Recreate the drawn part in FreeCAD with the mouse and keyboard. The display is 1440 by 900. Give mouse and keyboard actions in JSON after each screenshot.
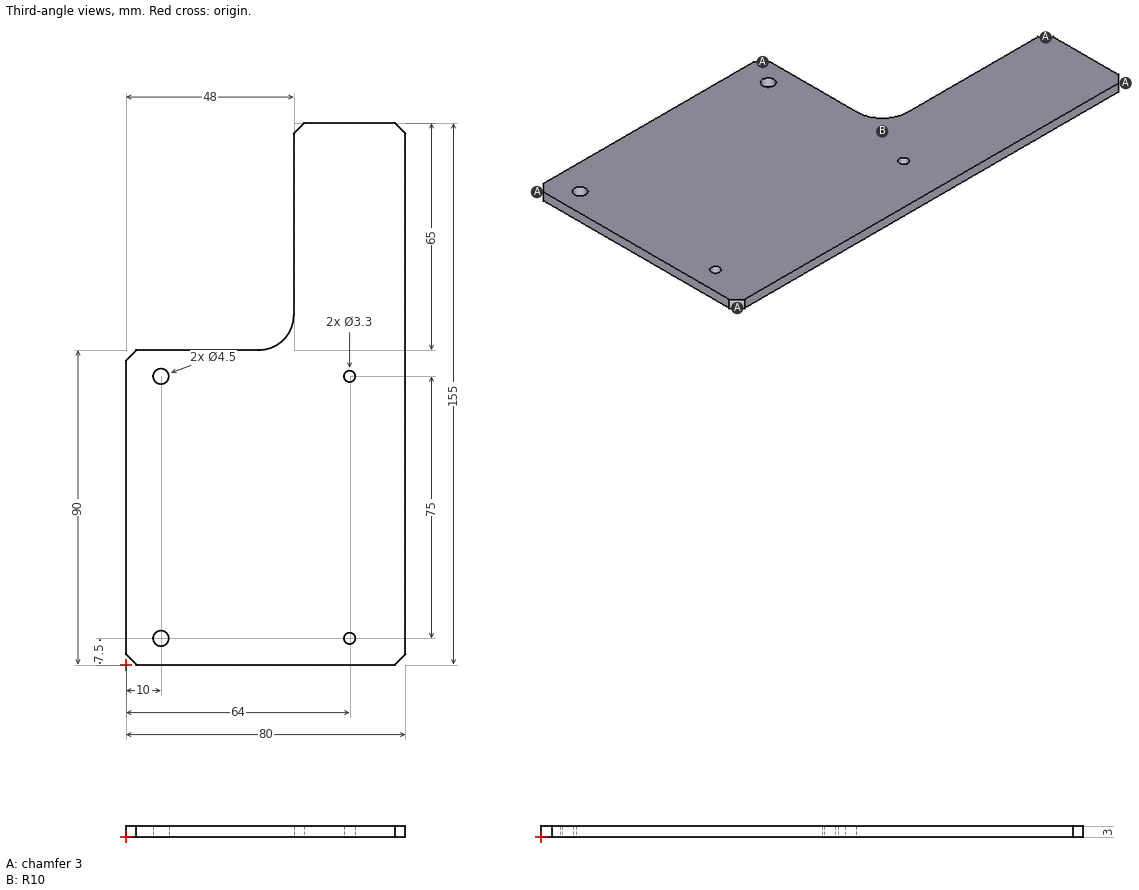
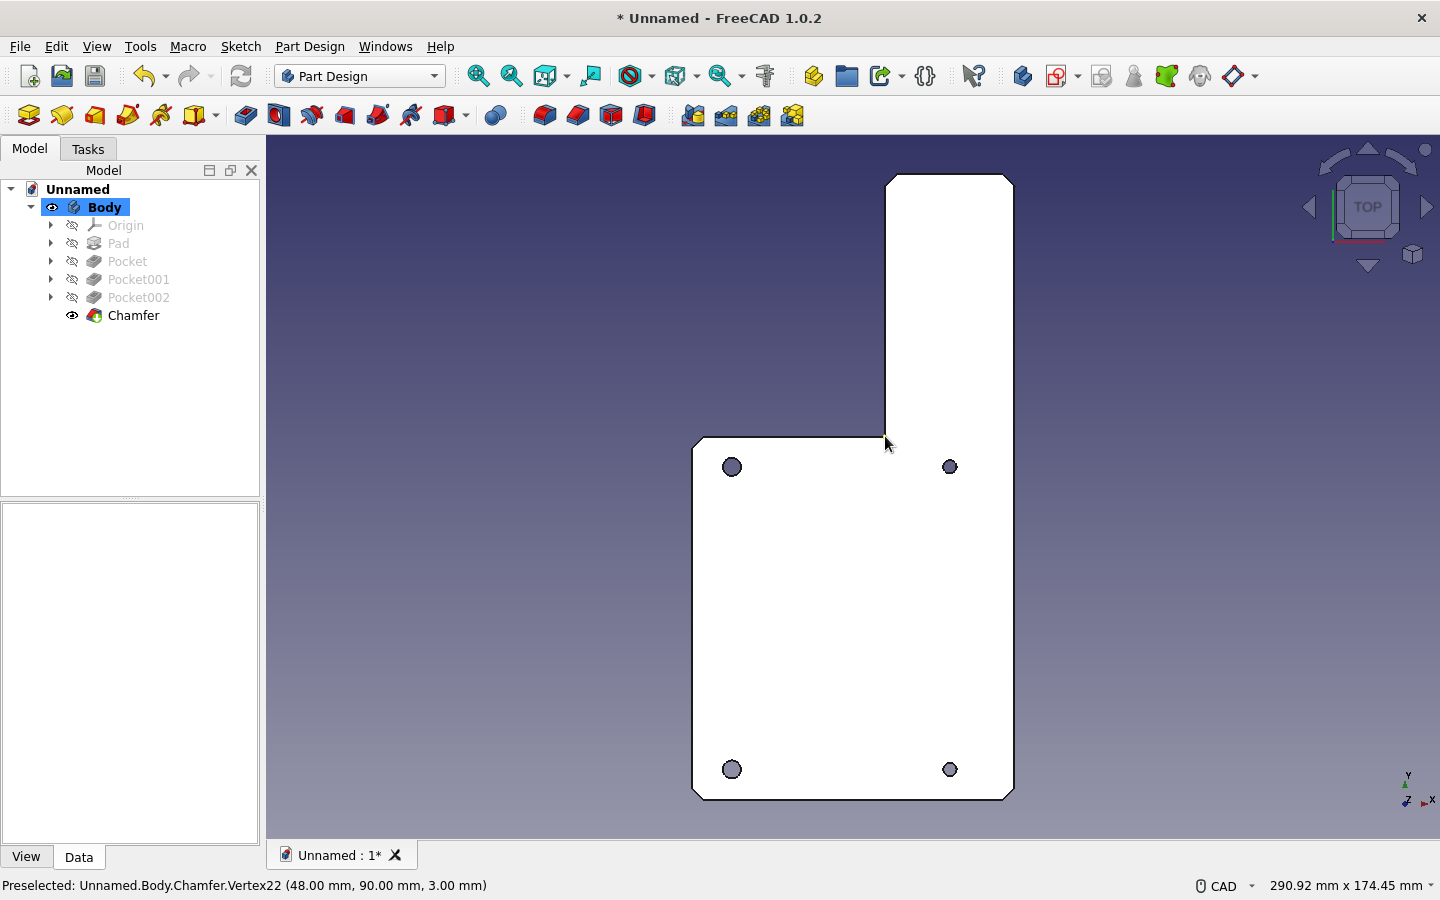
{"action": "key", "text": "1"}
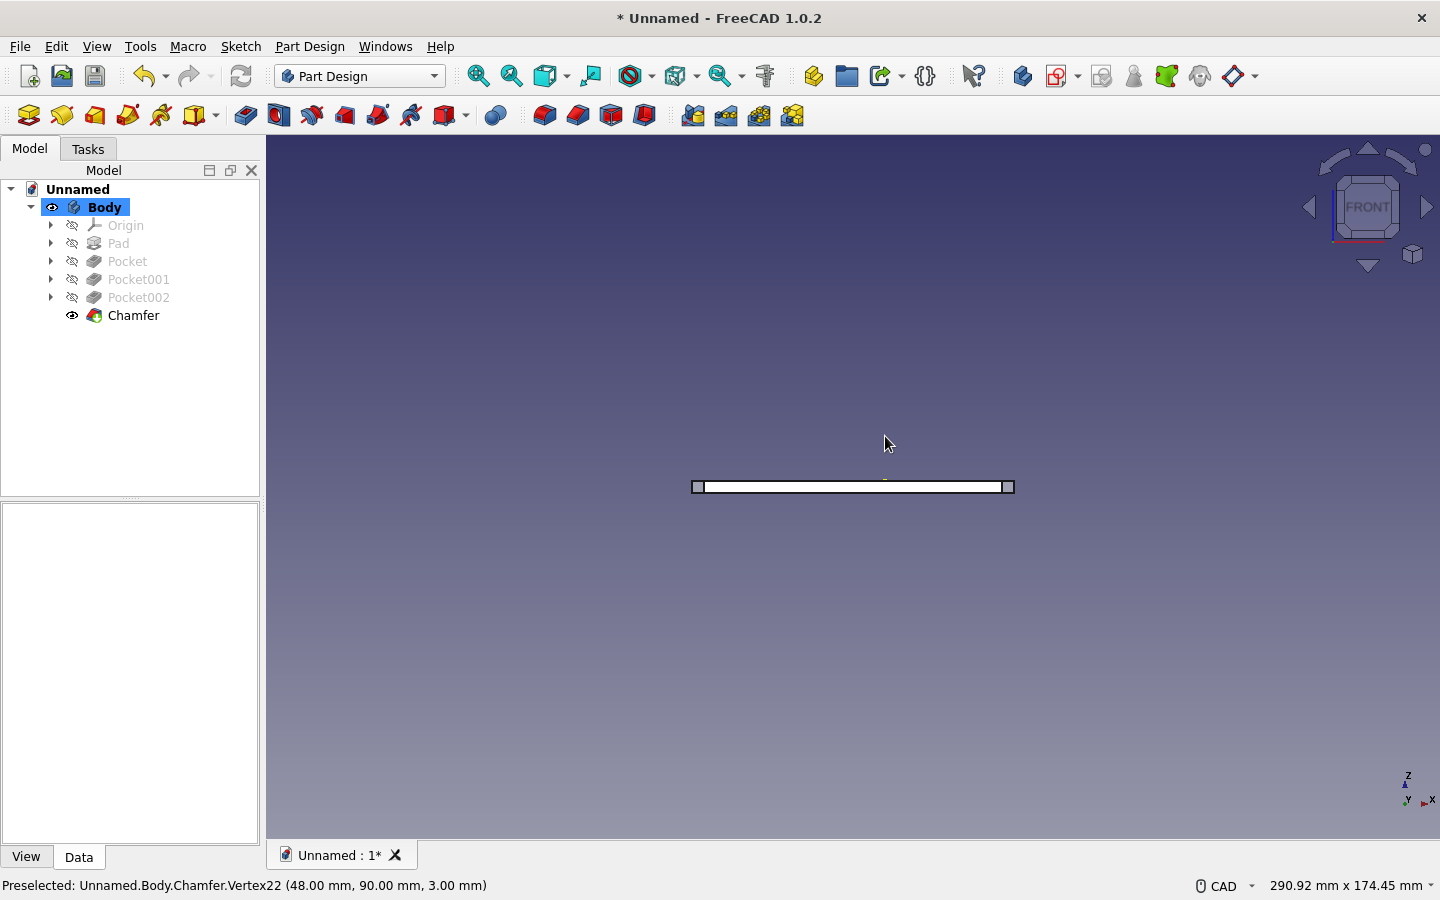
{"action": "key", "text": "v f"}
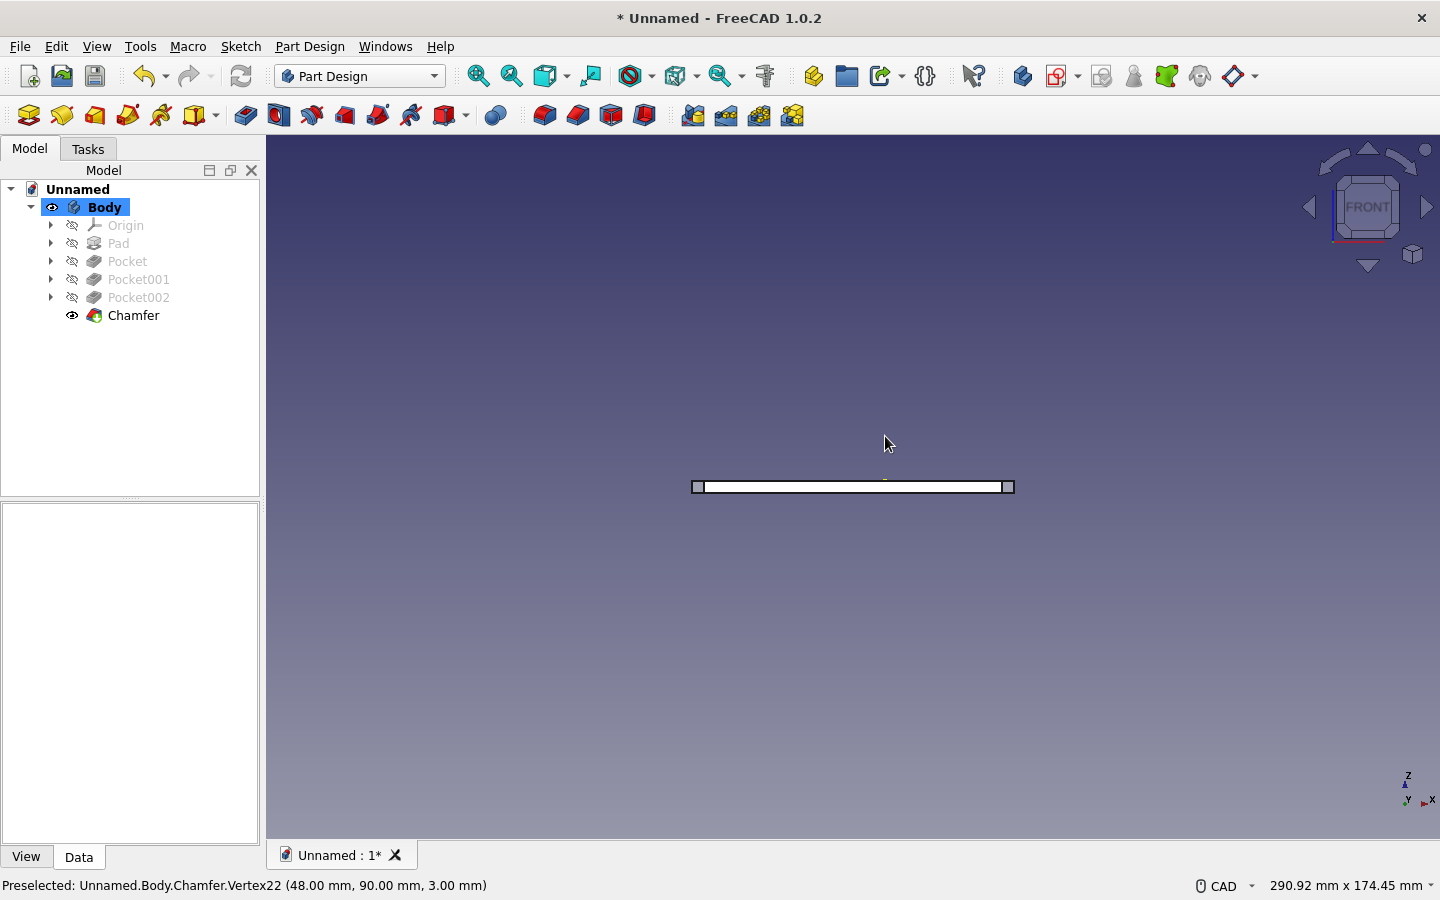
{"action": "scroll", "coordinate": [885, 486], "scroll_direction": "up", "scroll_amount": 6}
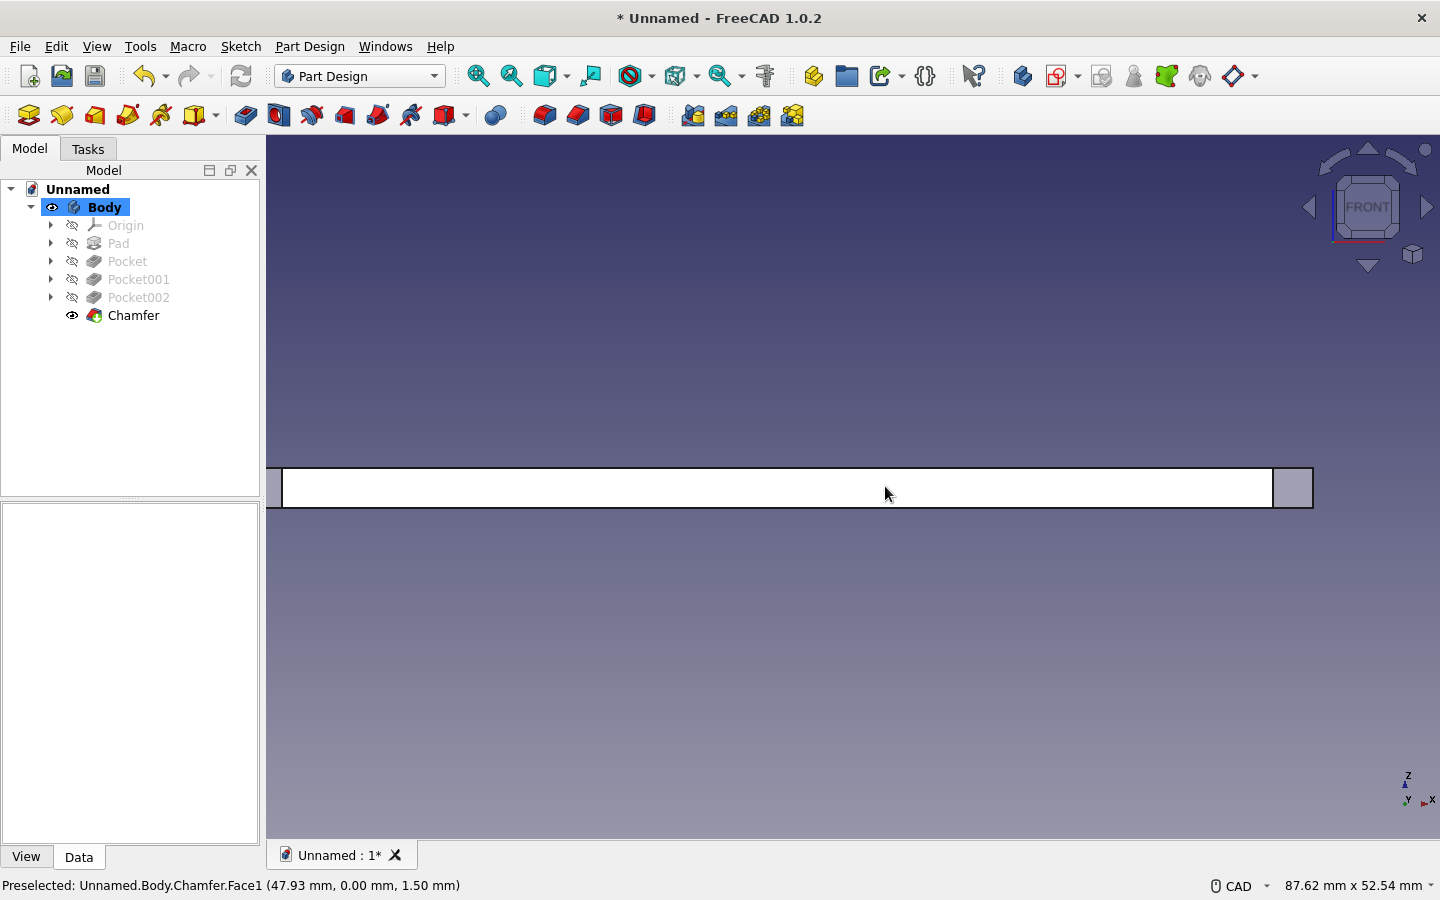
{"action": "left_click", "coordinate": [479, 76]}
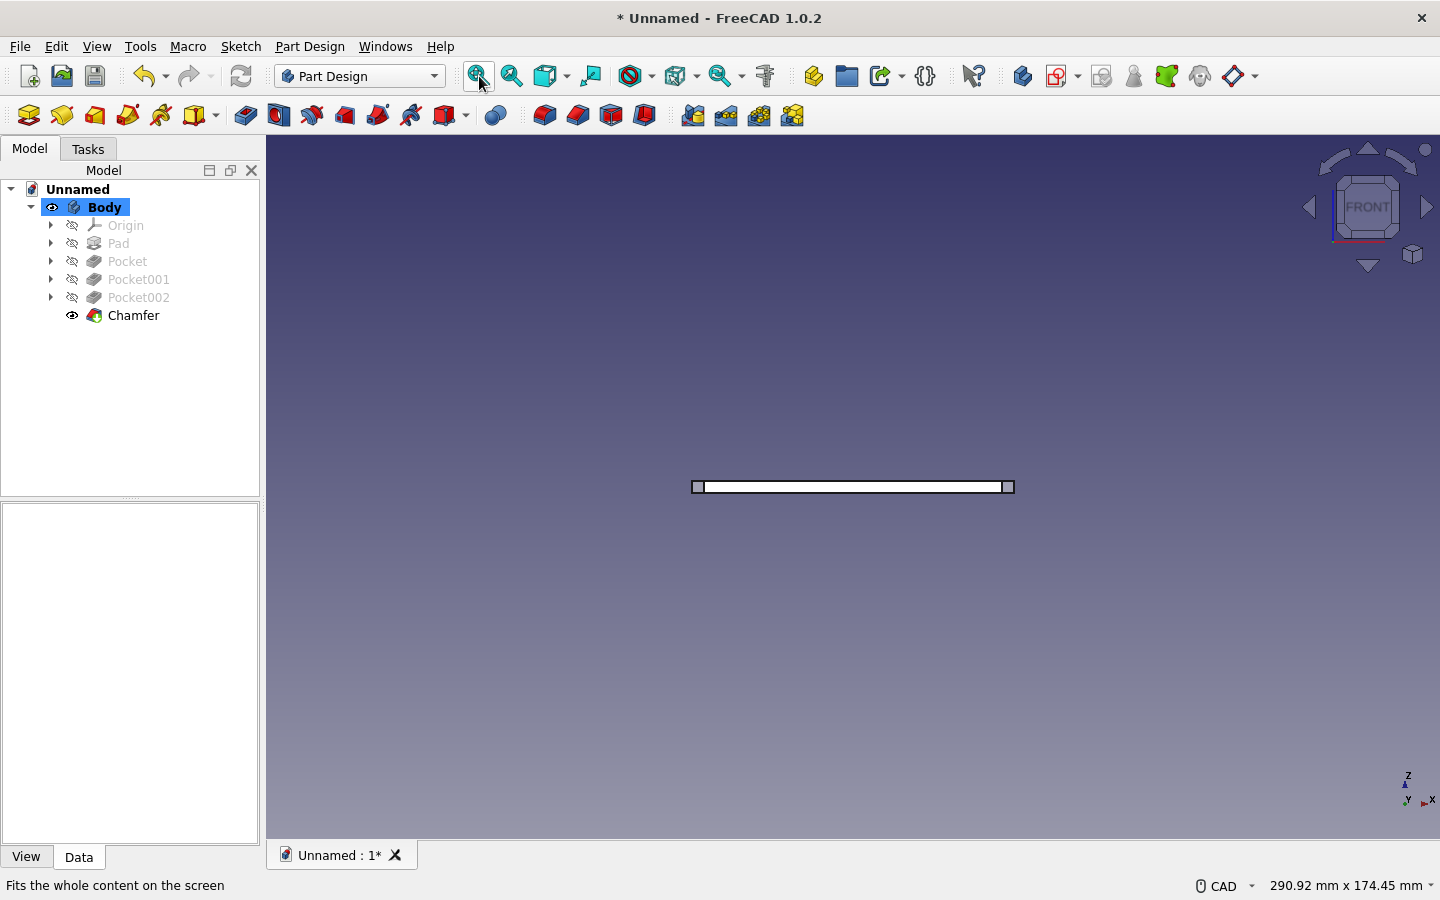
{"action": "key", "text": "3"}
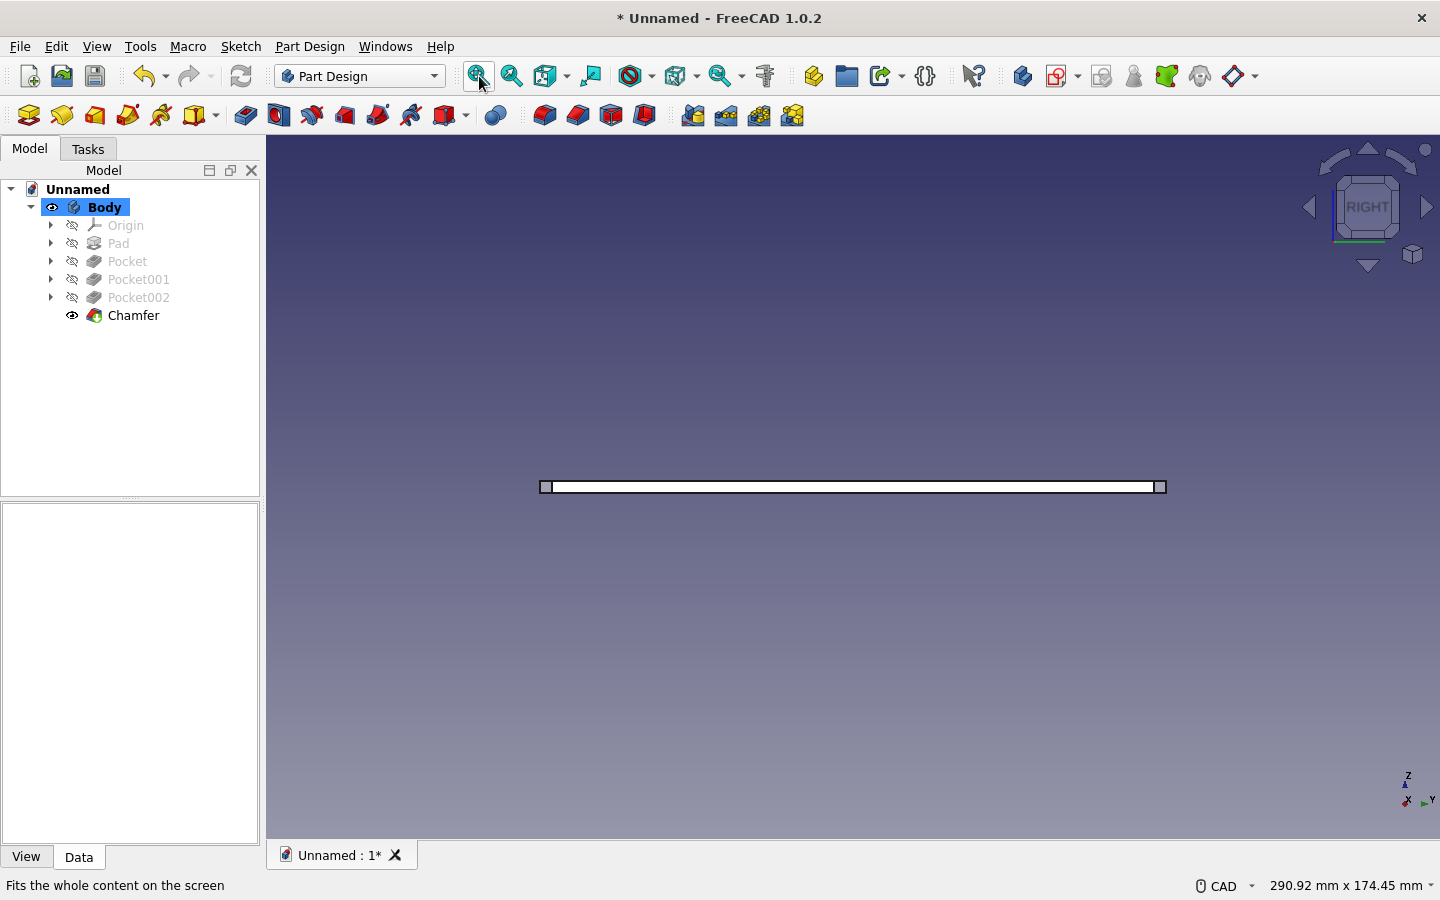
{"action": "scroll", "coordinate": [903, 486], "scroll_direction": "up", "scroll_amount": 6}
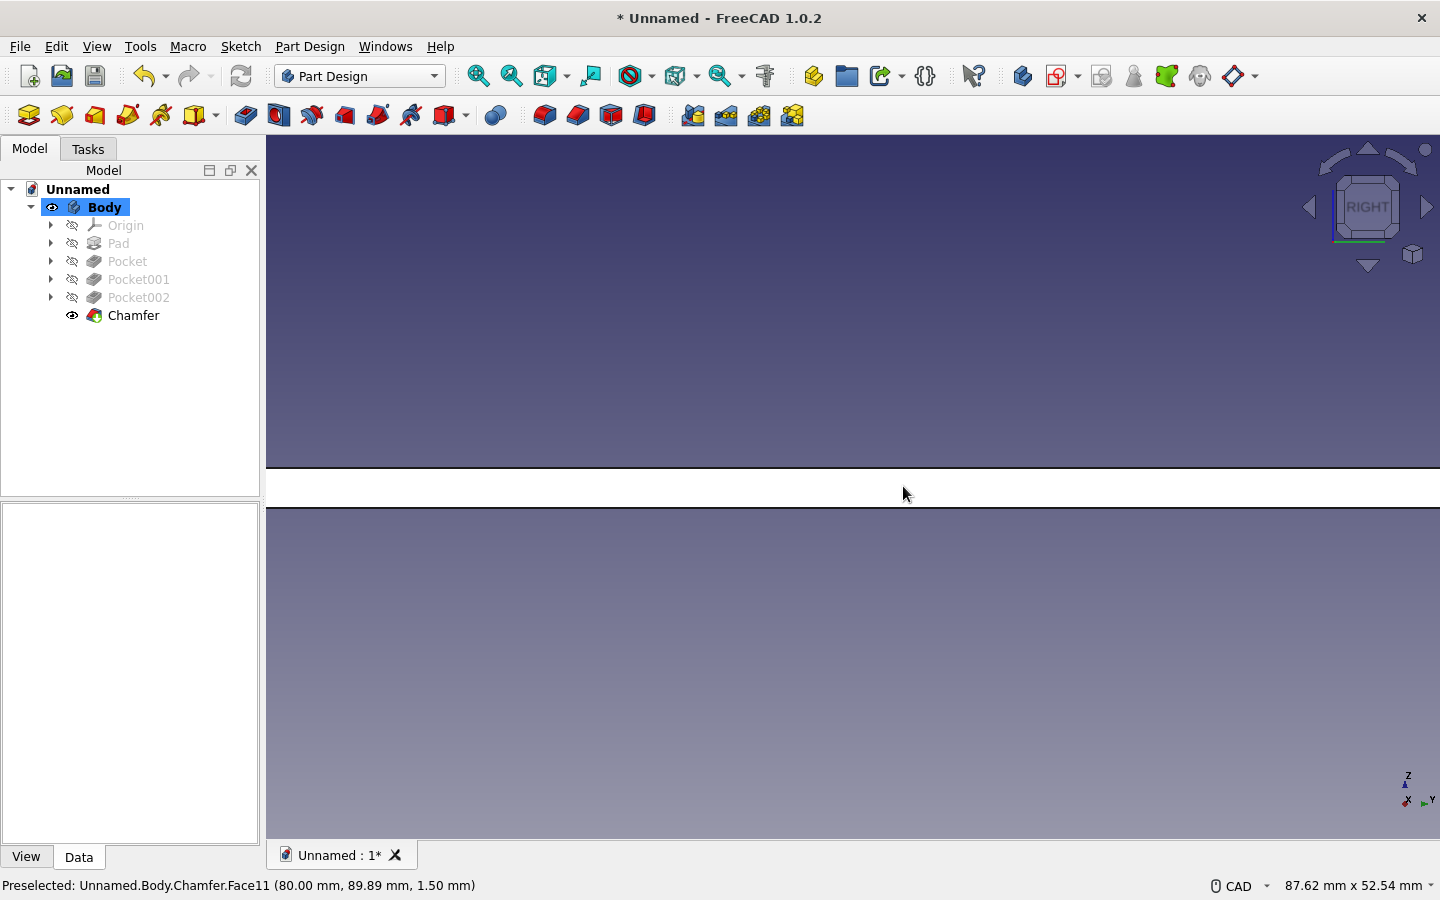
{"action": "key", "text": "v f"}